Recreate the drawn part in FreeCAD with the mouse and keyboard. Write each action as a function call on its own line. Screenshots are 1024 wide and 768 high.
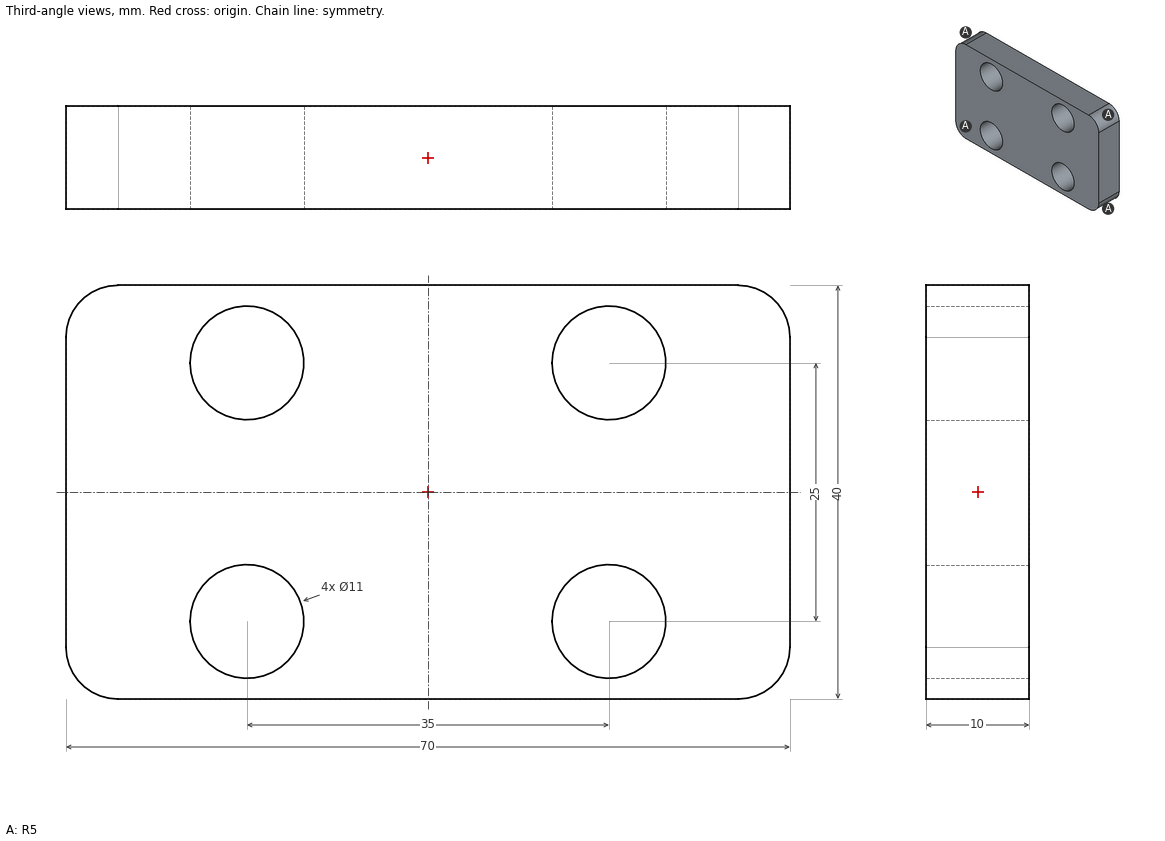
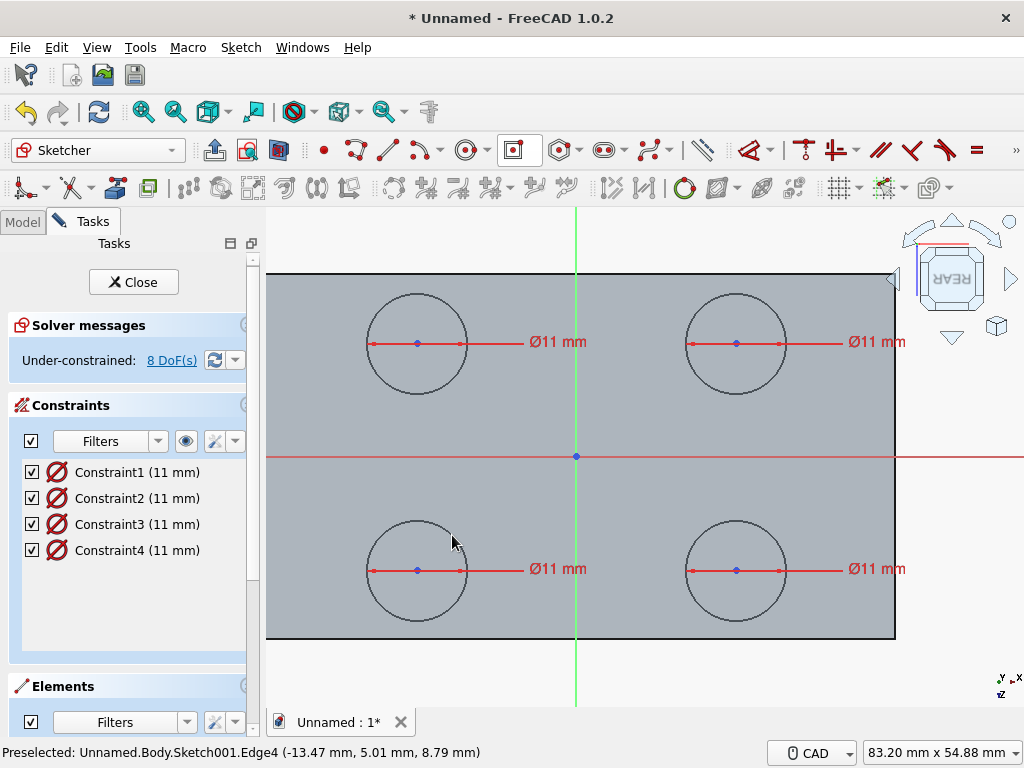
click(417, 344)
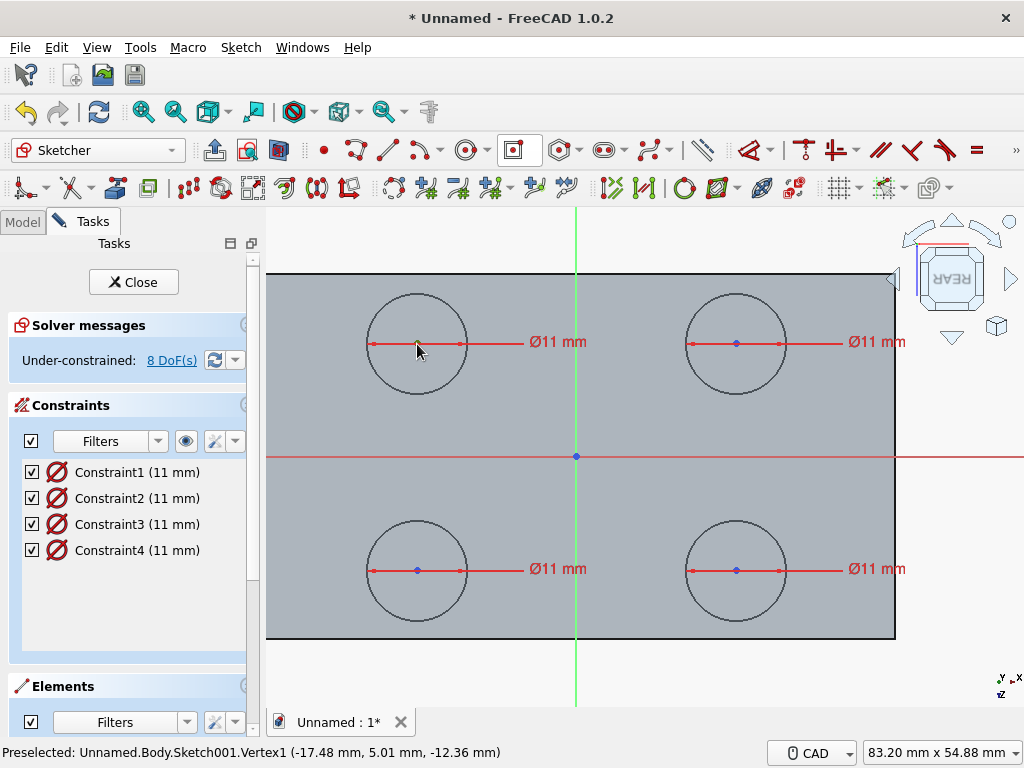
click(736, 344)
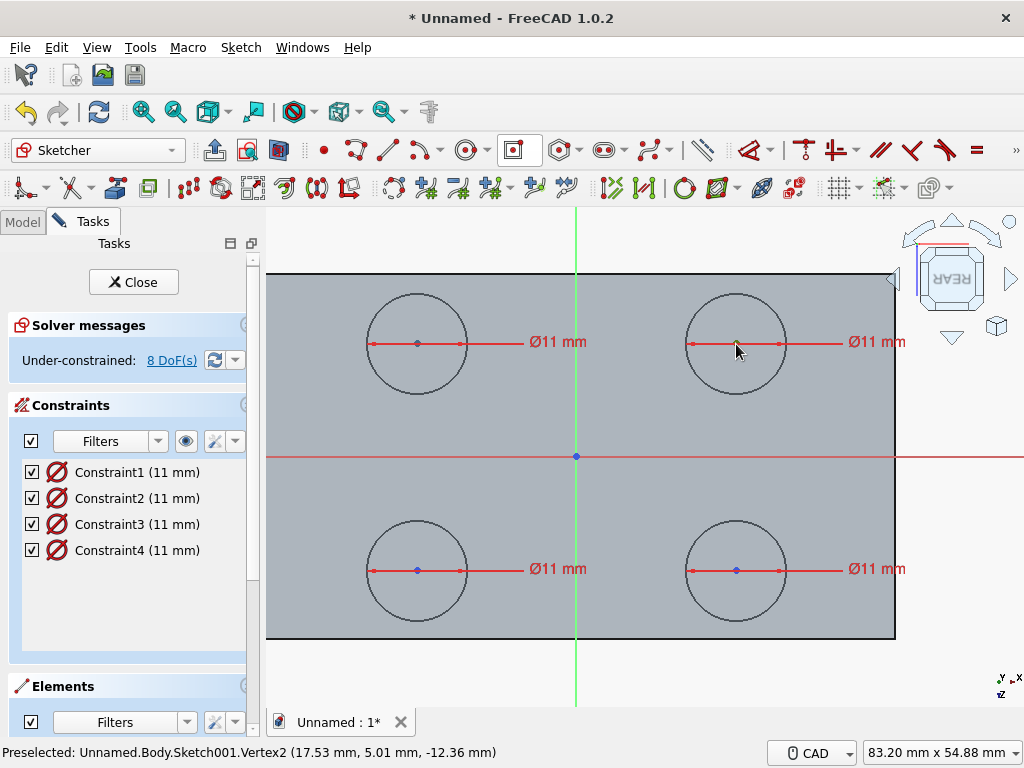
click(576, 647)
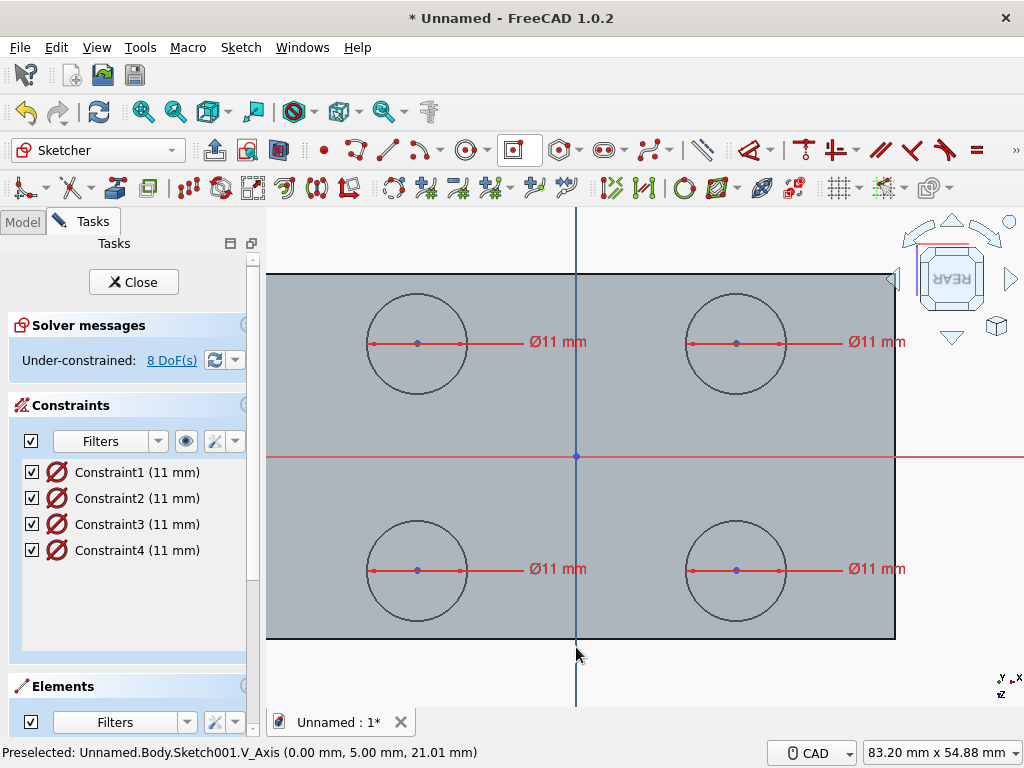
key(s)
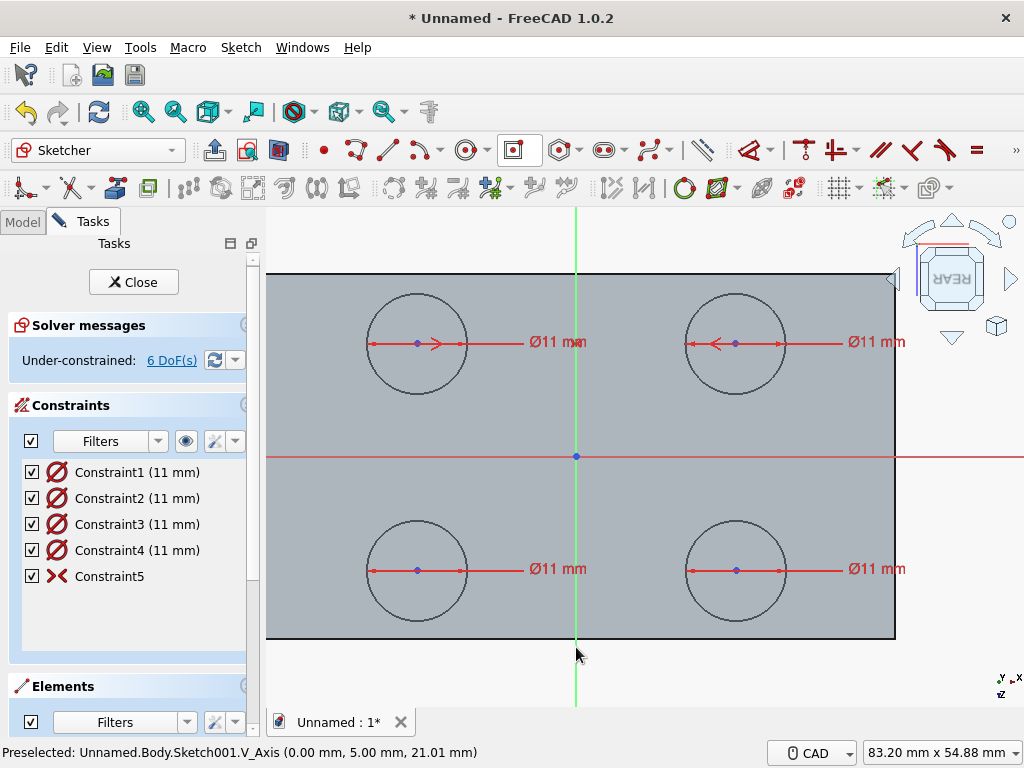
click(736, 344)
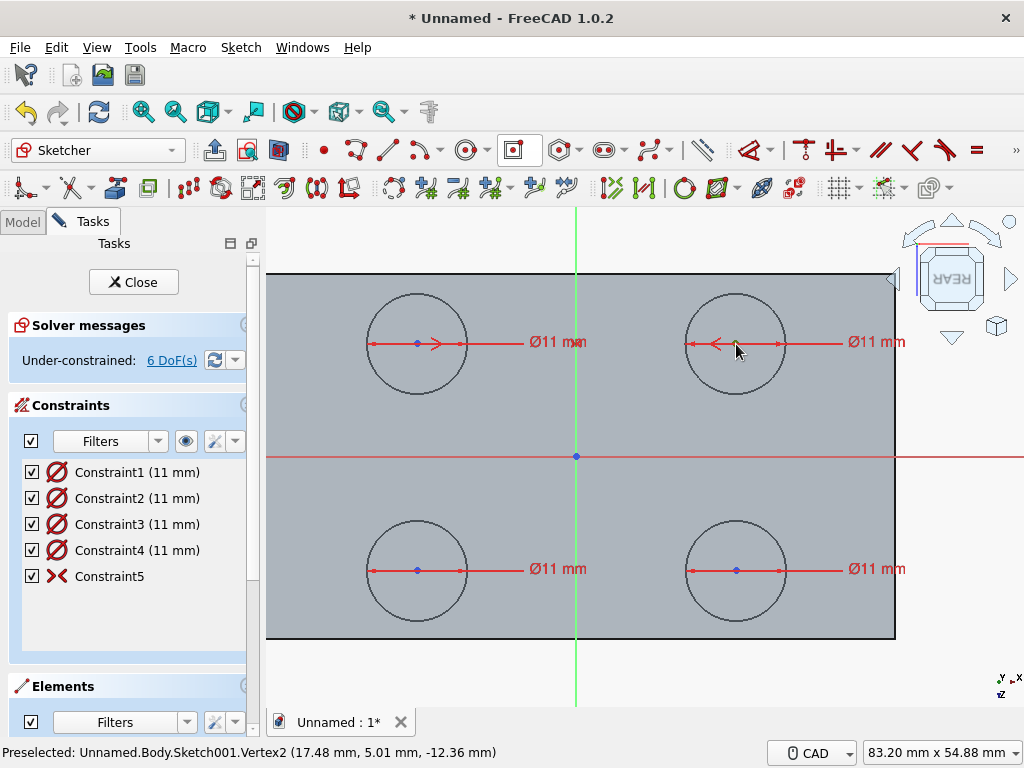
click(736, 571)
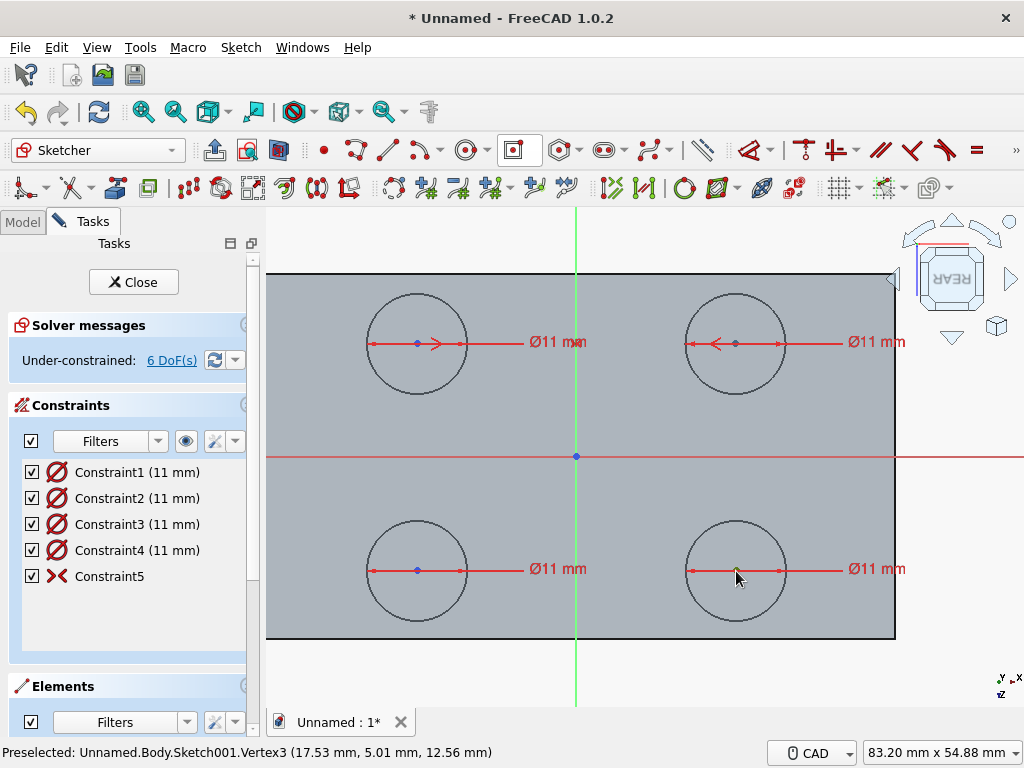
click(334, 457)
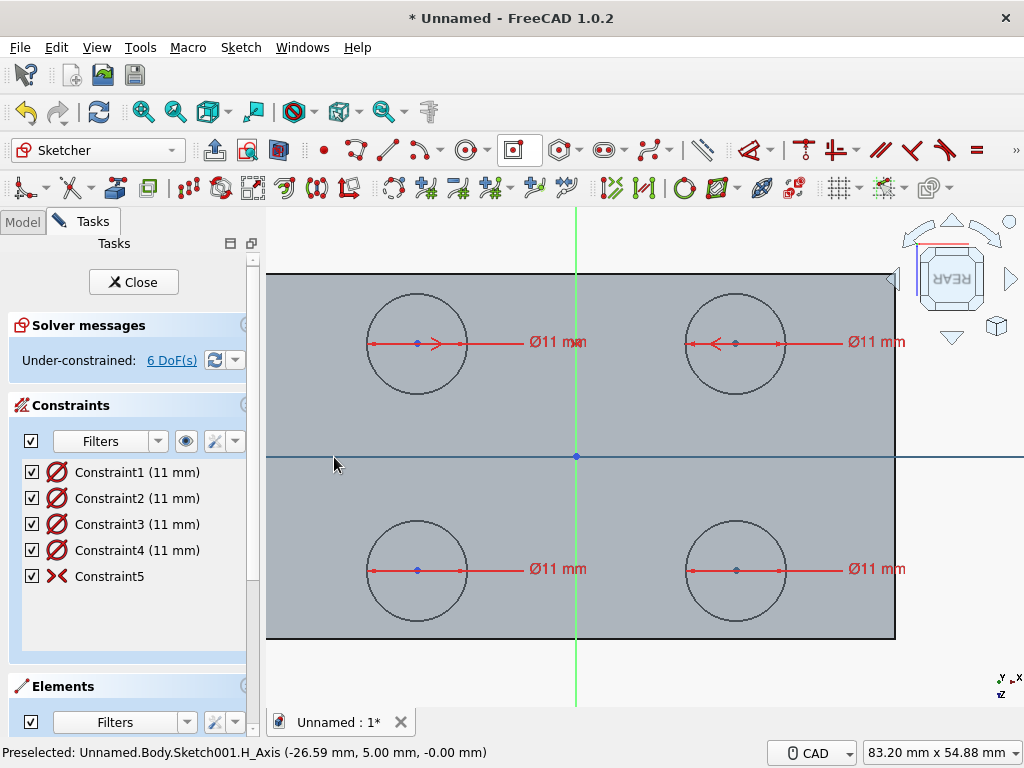
key(s)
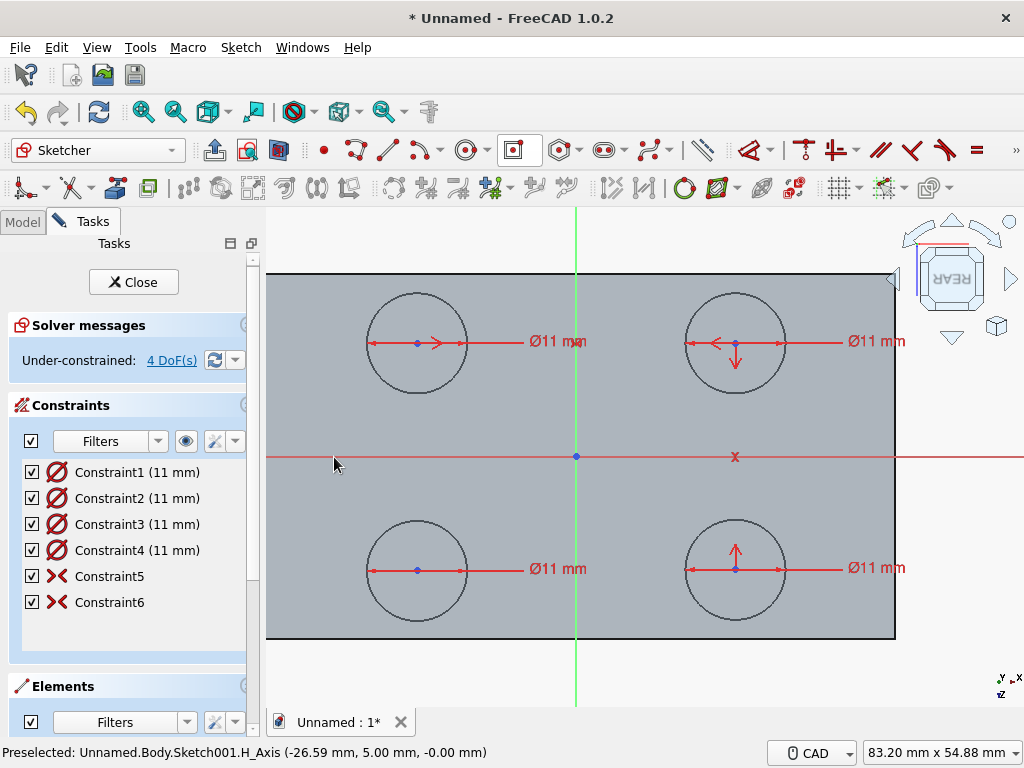
click(417, 343)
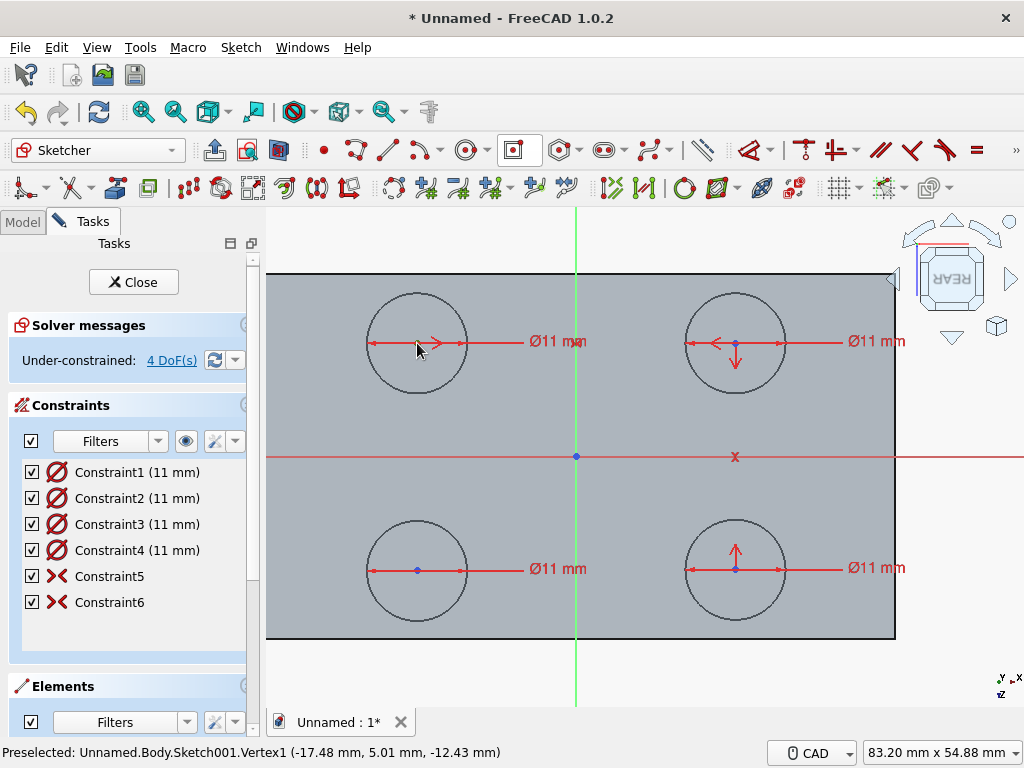
click(417, 571)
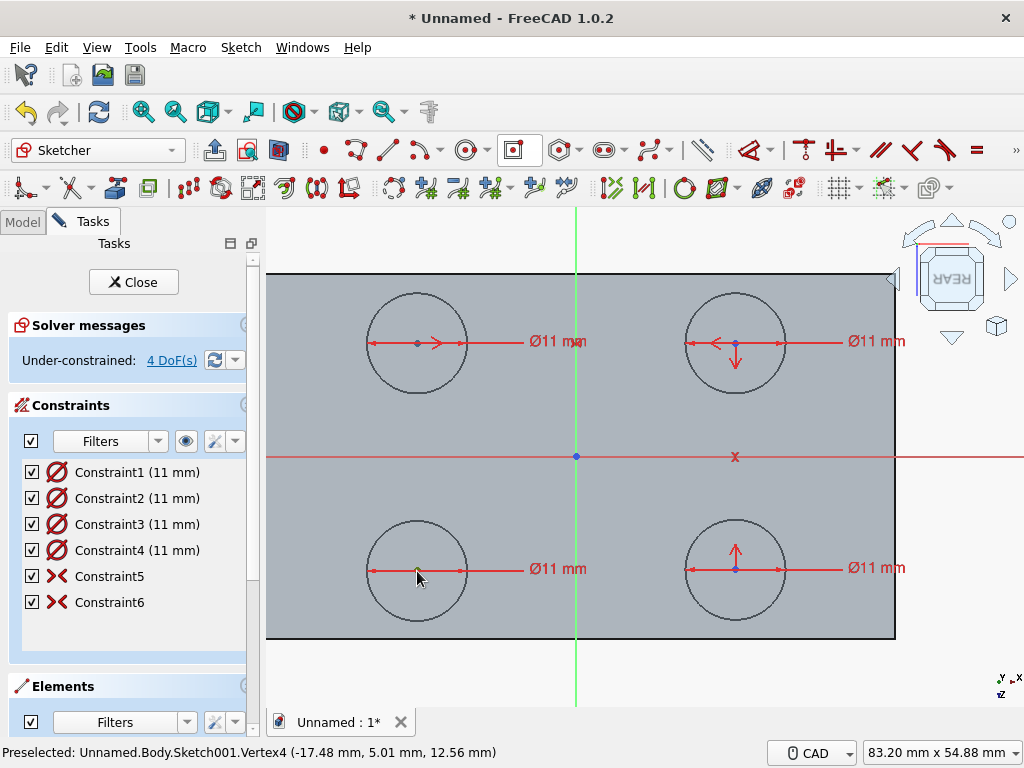
click(334, 457)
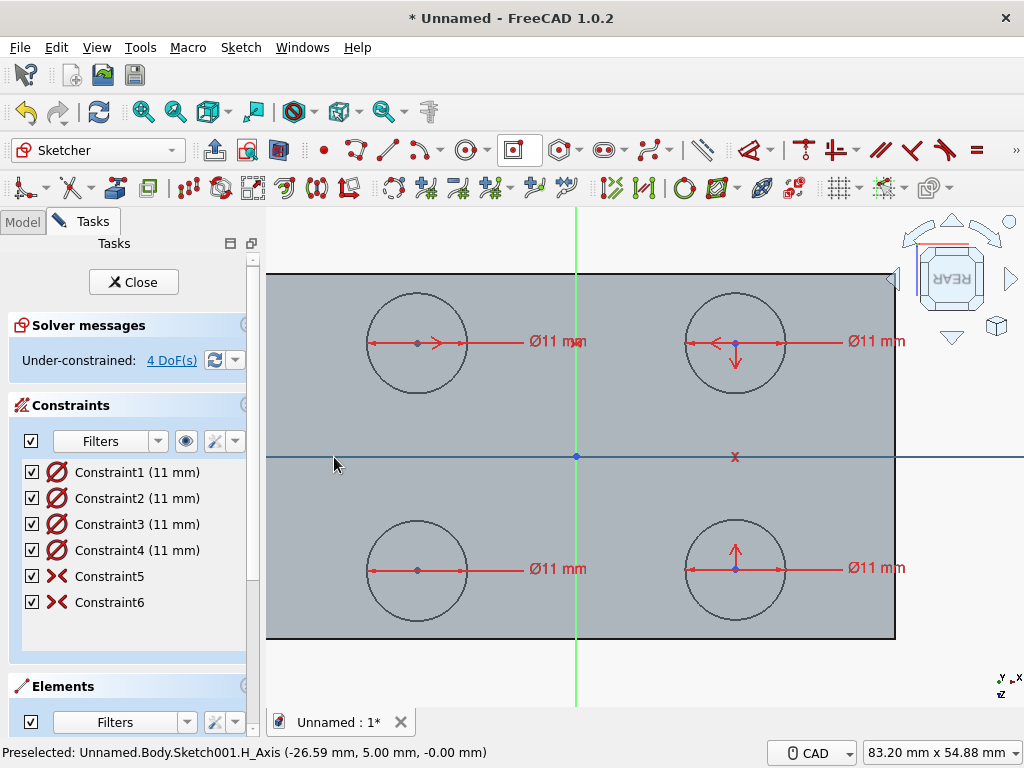
key(s)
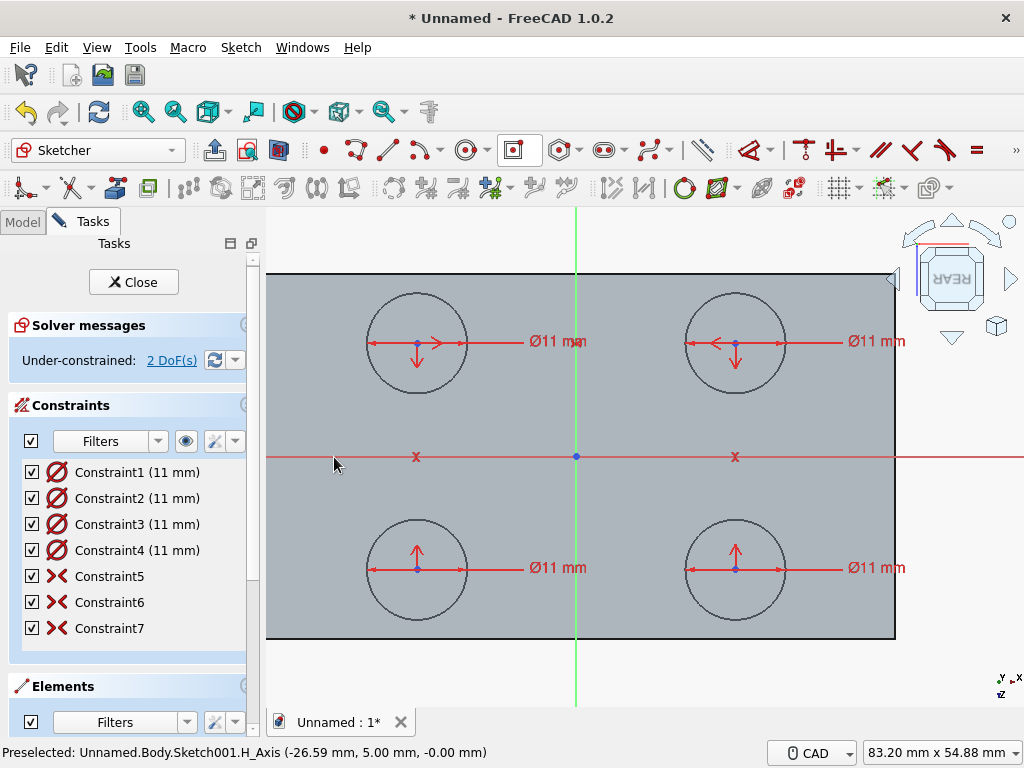
key(d)